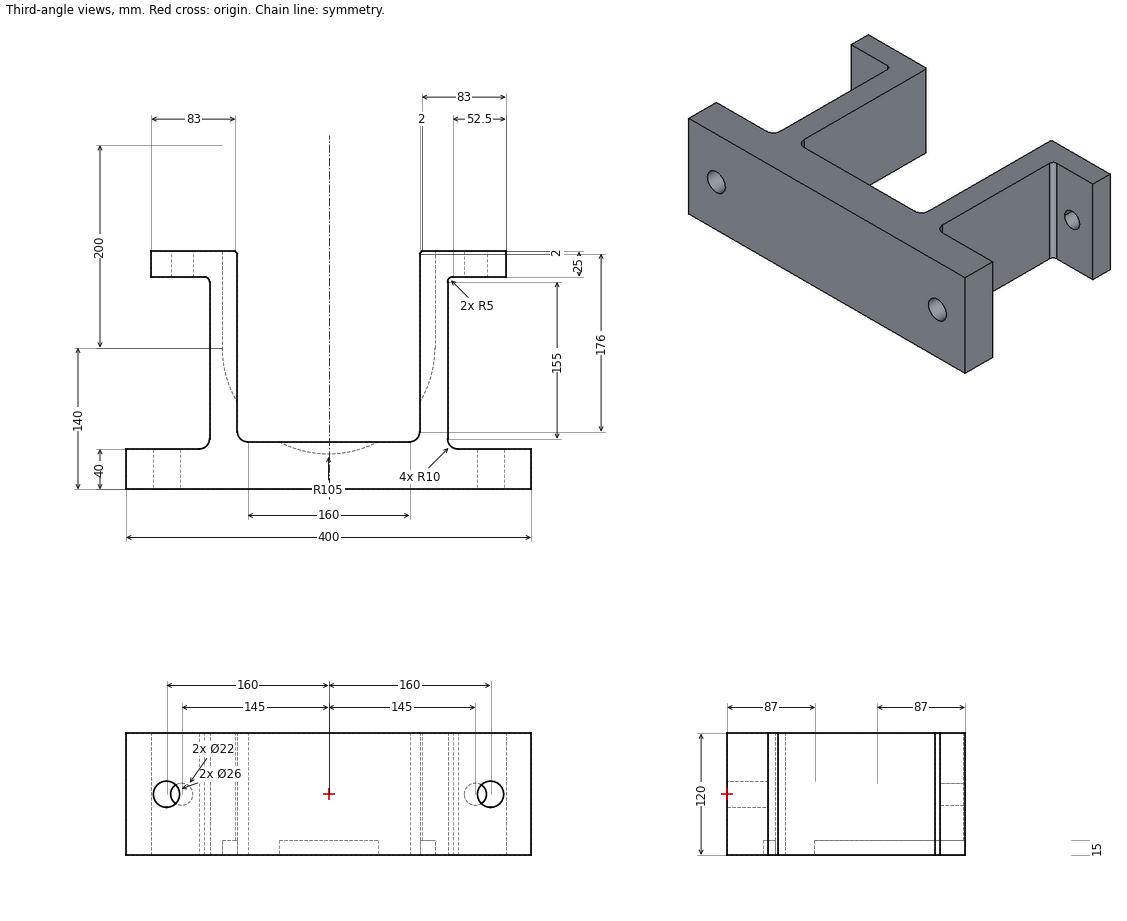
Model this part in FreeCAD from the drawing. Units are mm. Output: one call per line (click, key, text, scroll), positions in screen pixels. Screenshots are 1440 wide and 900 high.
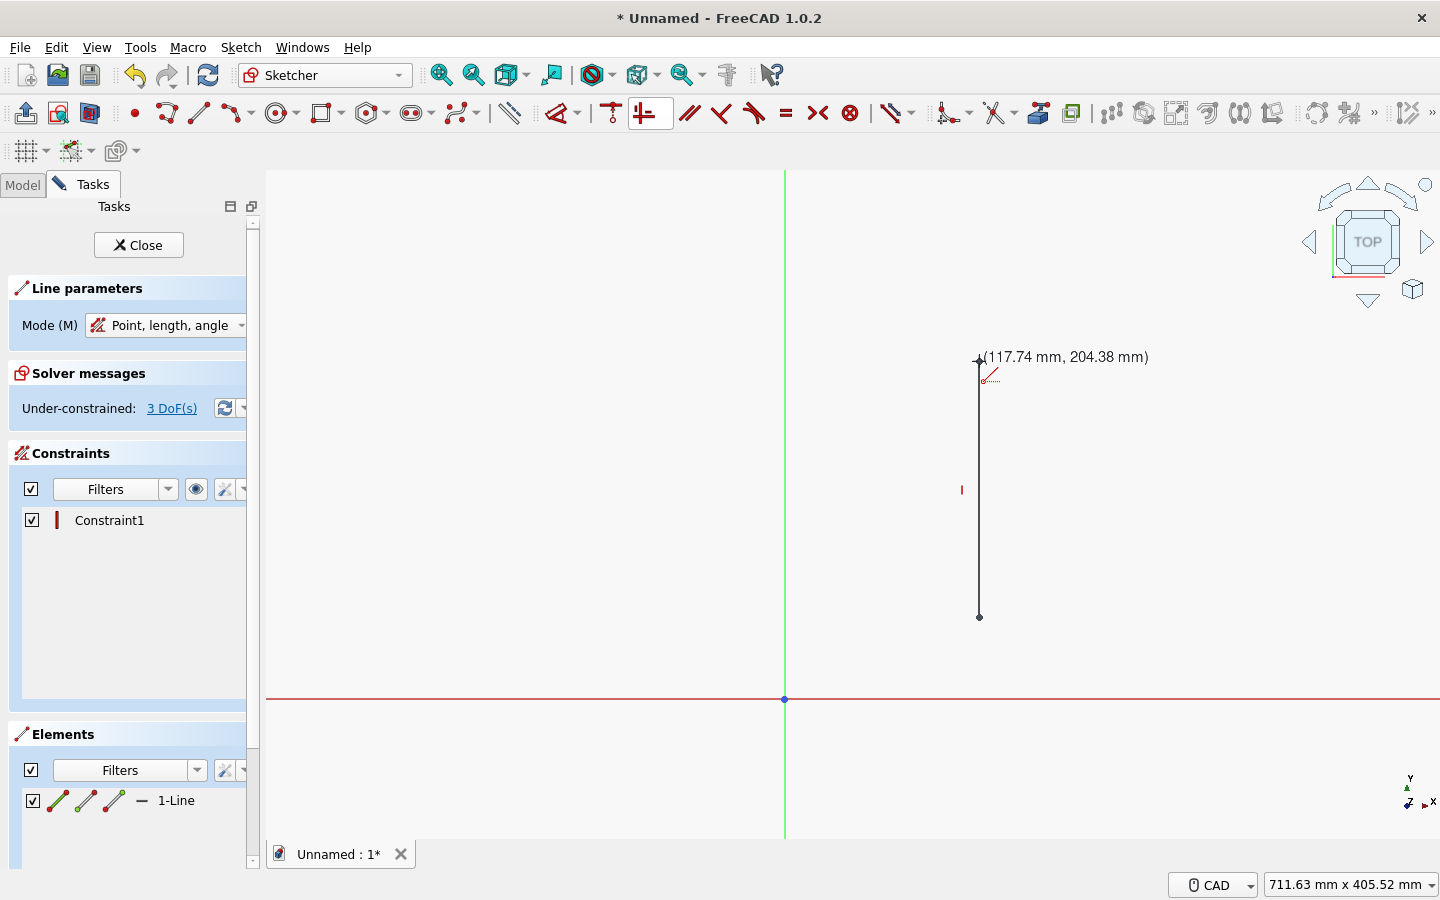
click(168, 114)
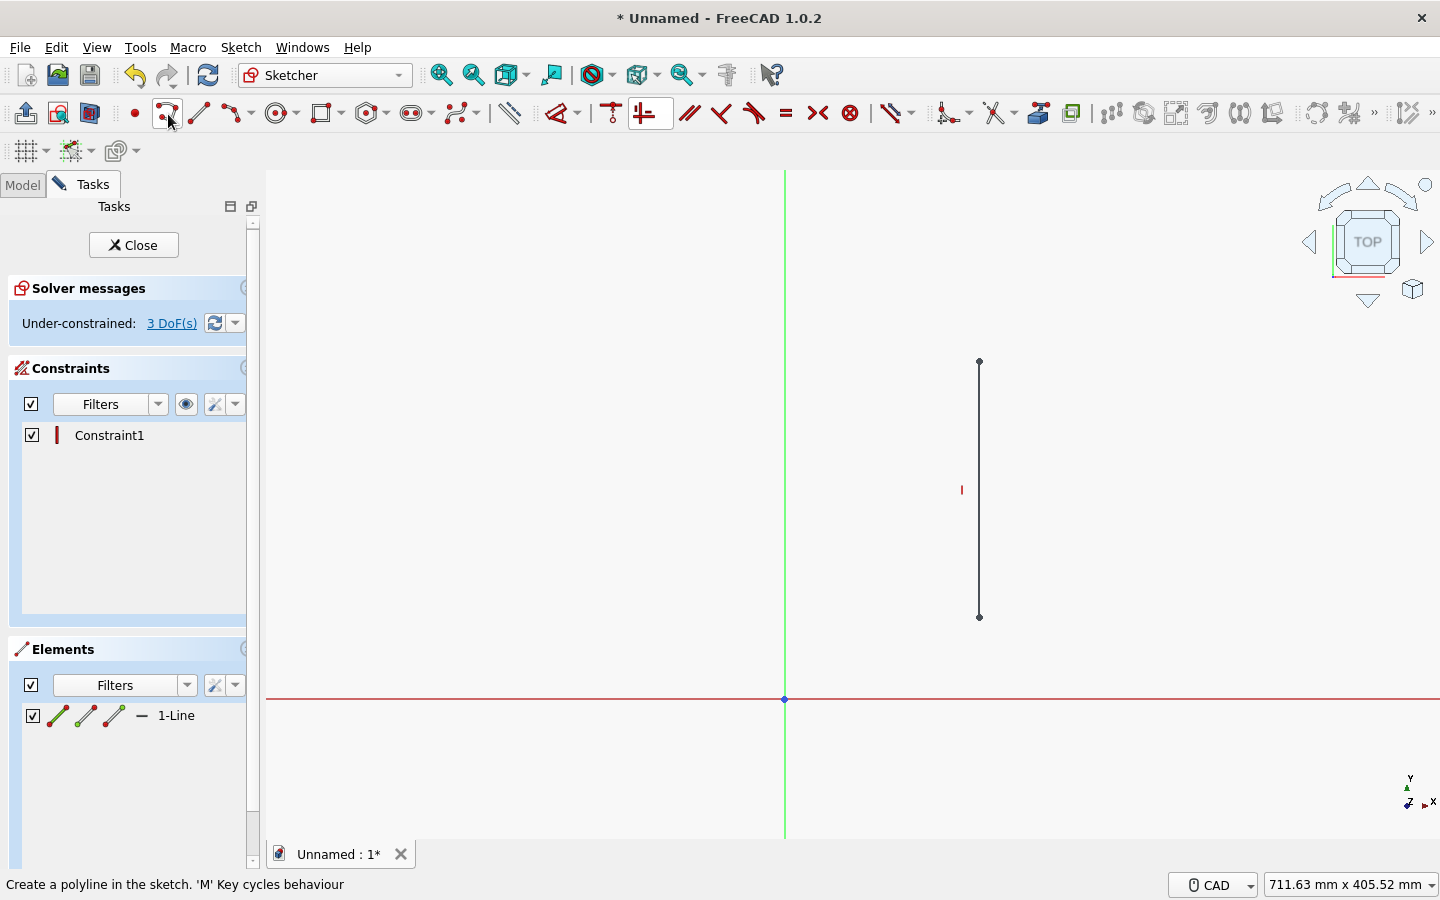
scroll(987, 353, up, 2)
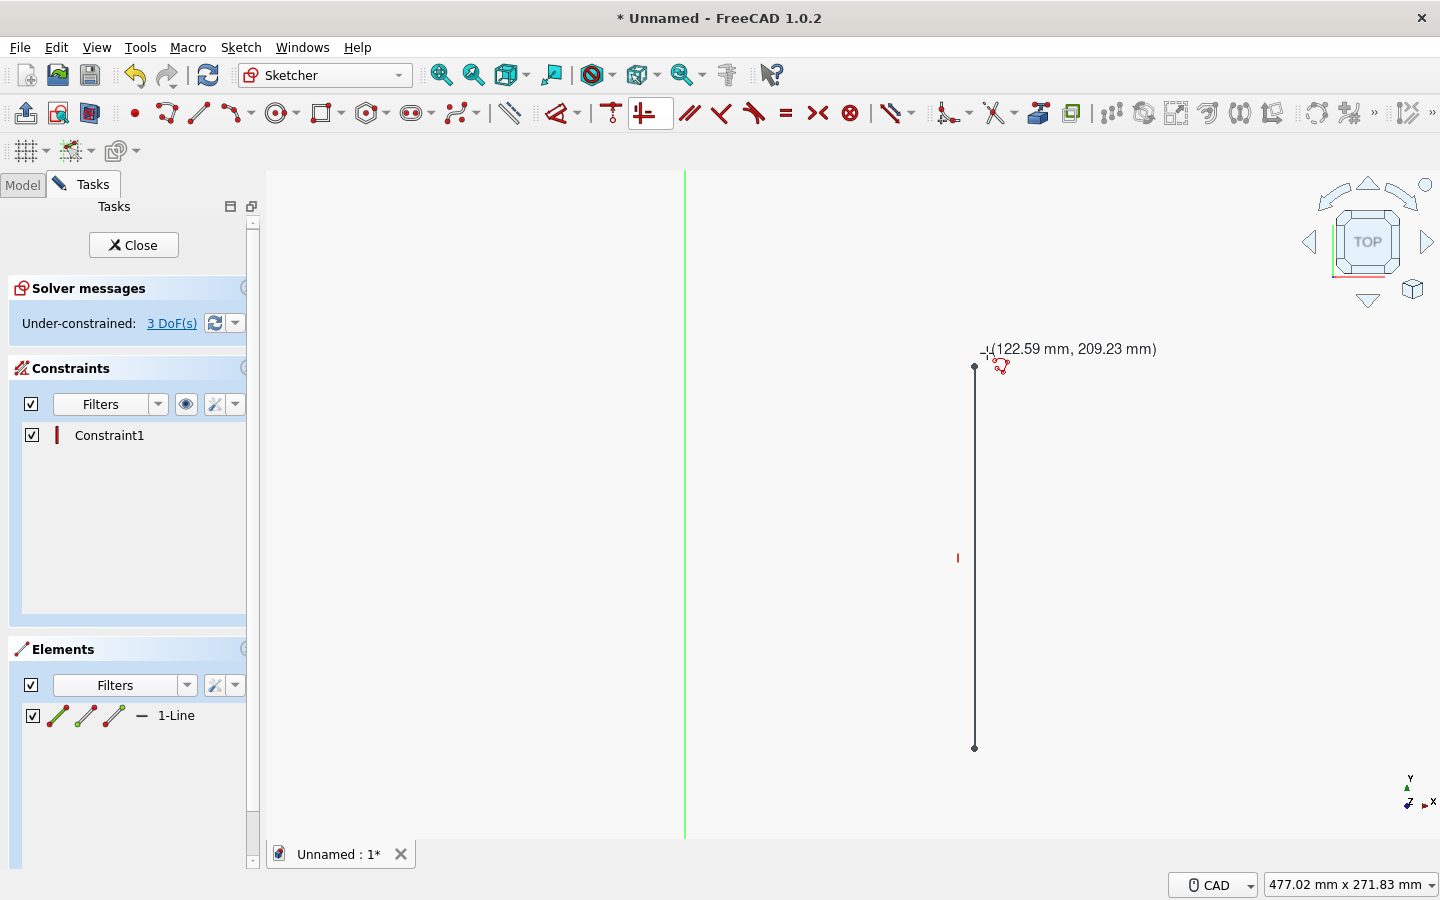
click(986, 352)
click(1116, 352)
click(1116, 291)
click(911, 291)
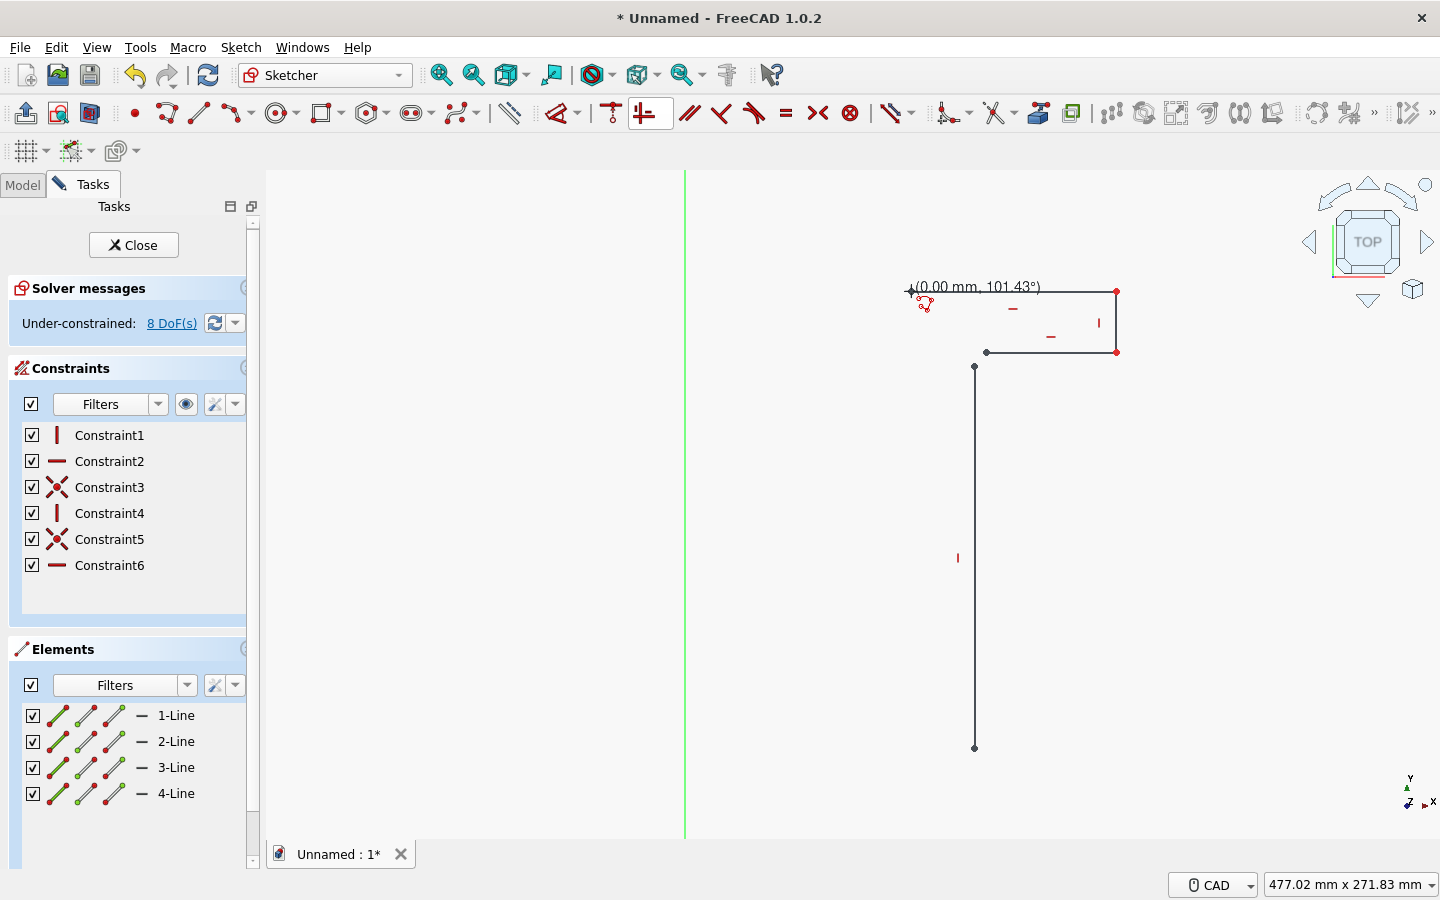
scroll(906, 296, up, 5)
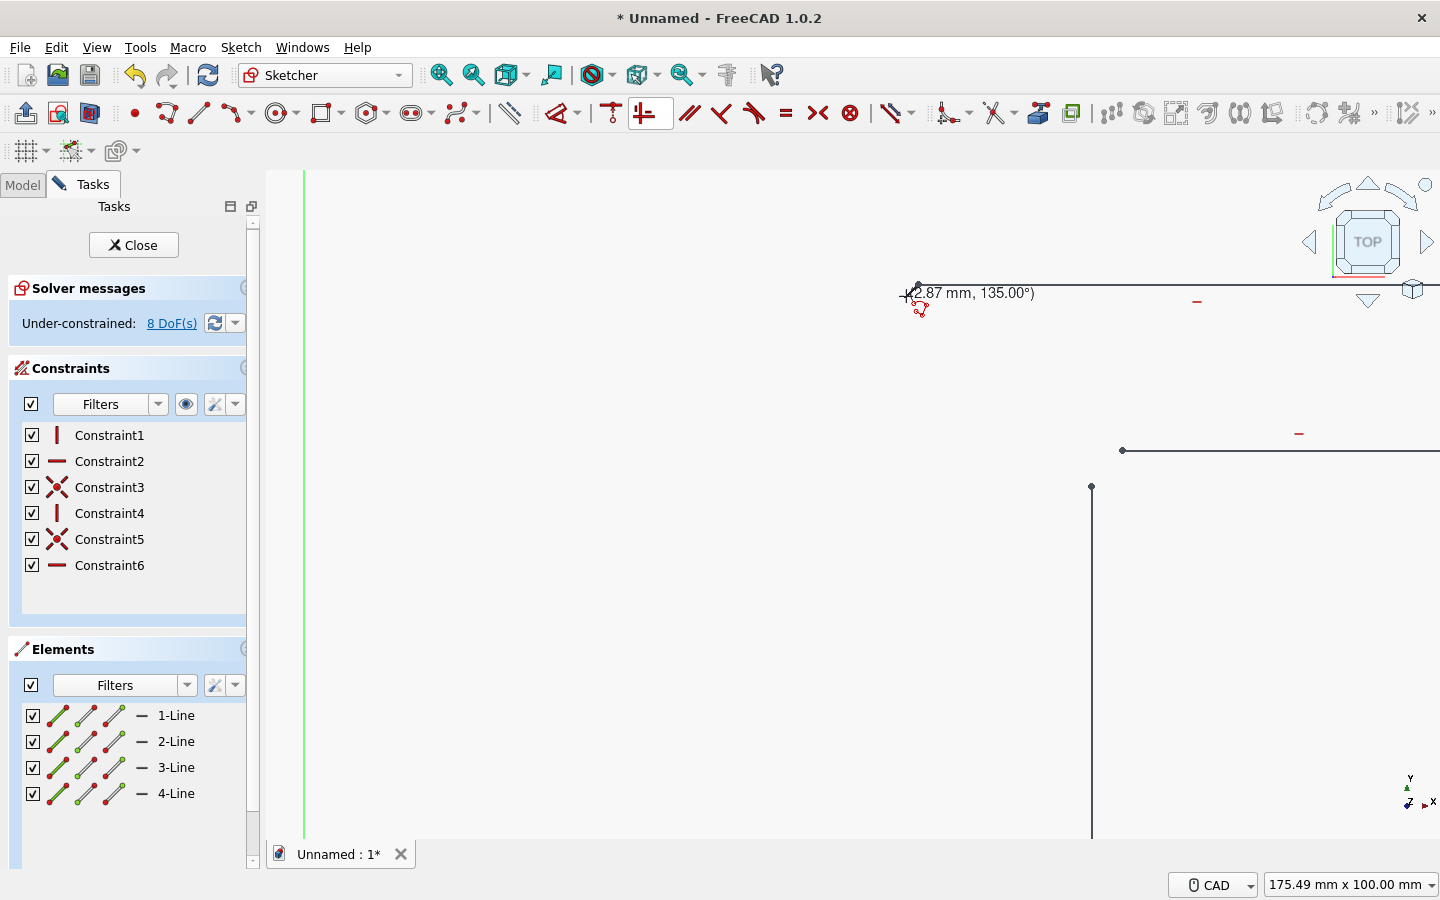
click(906, 295)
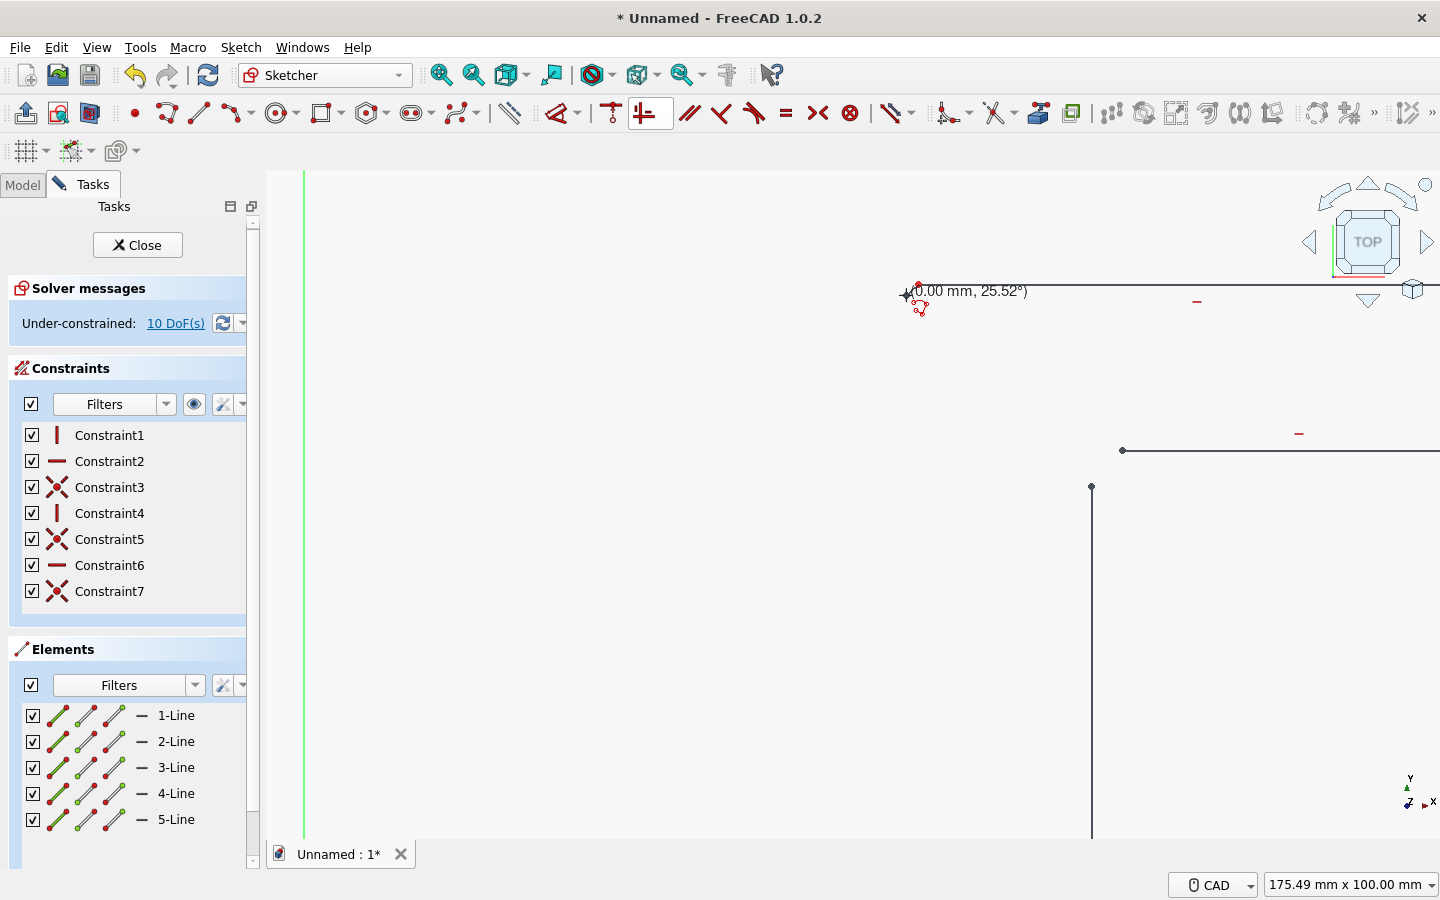
scroll(942, 320, down, 7)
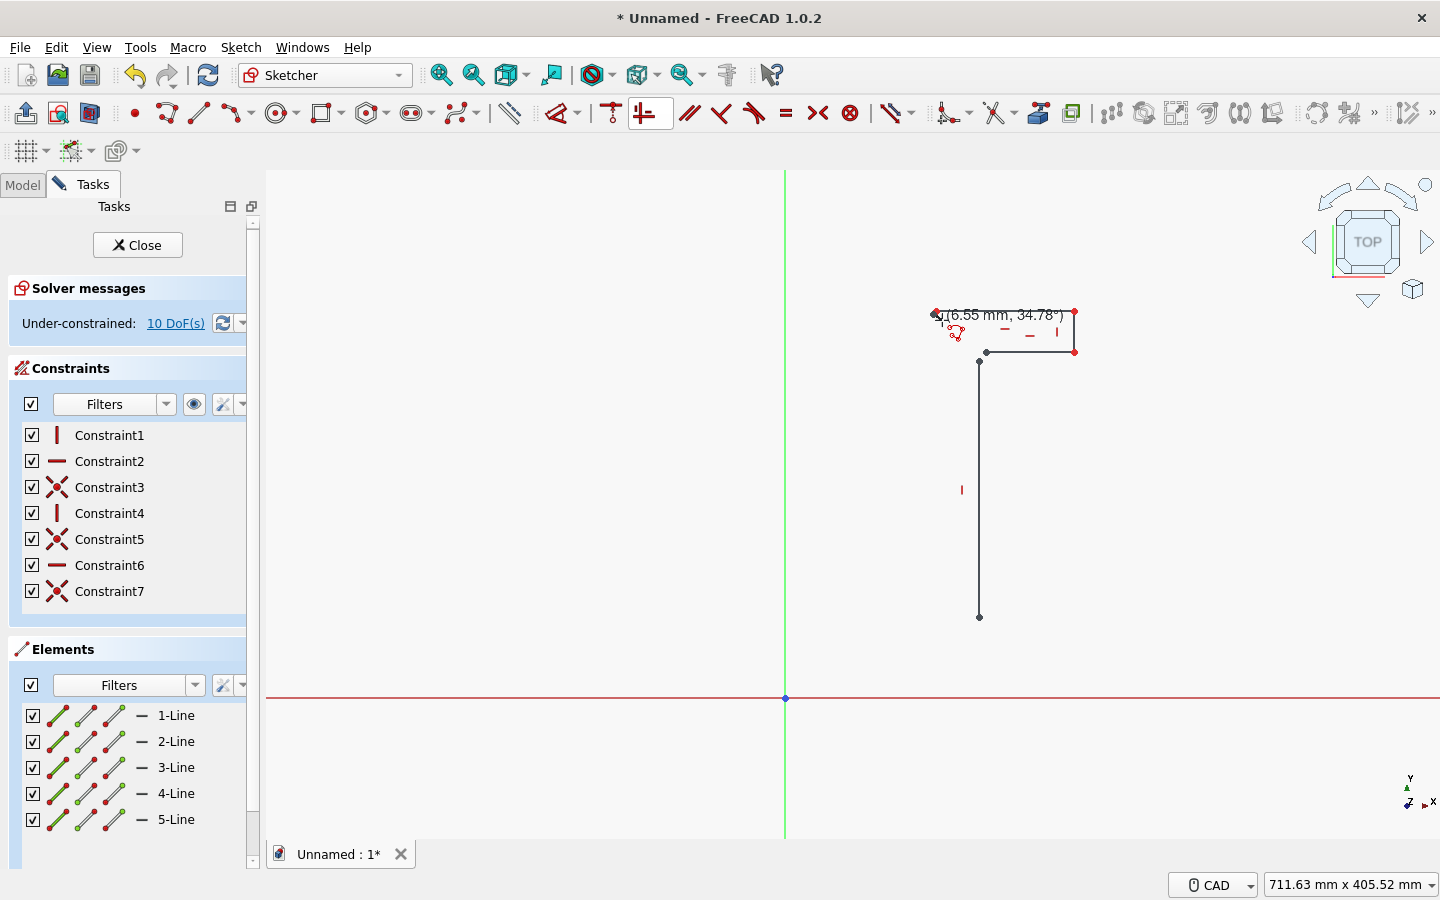
click(934, 604)
right_click(934, 604)